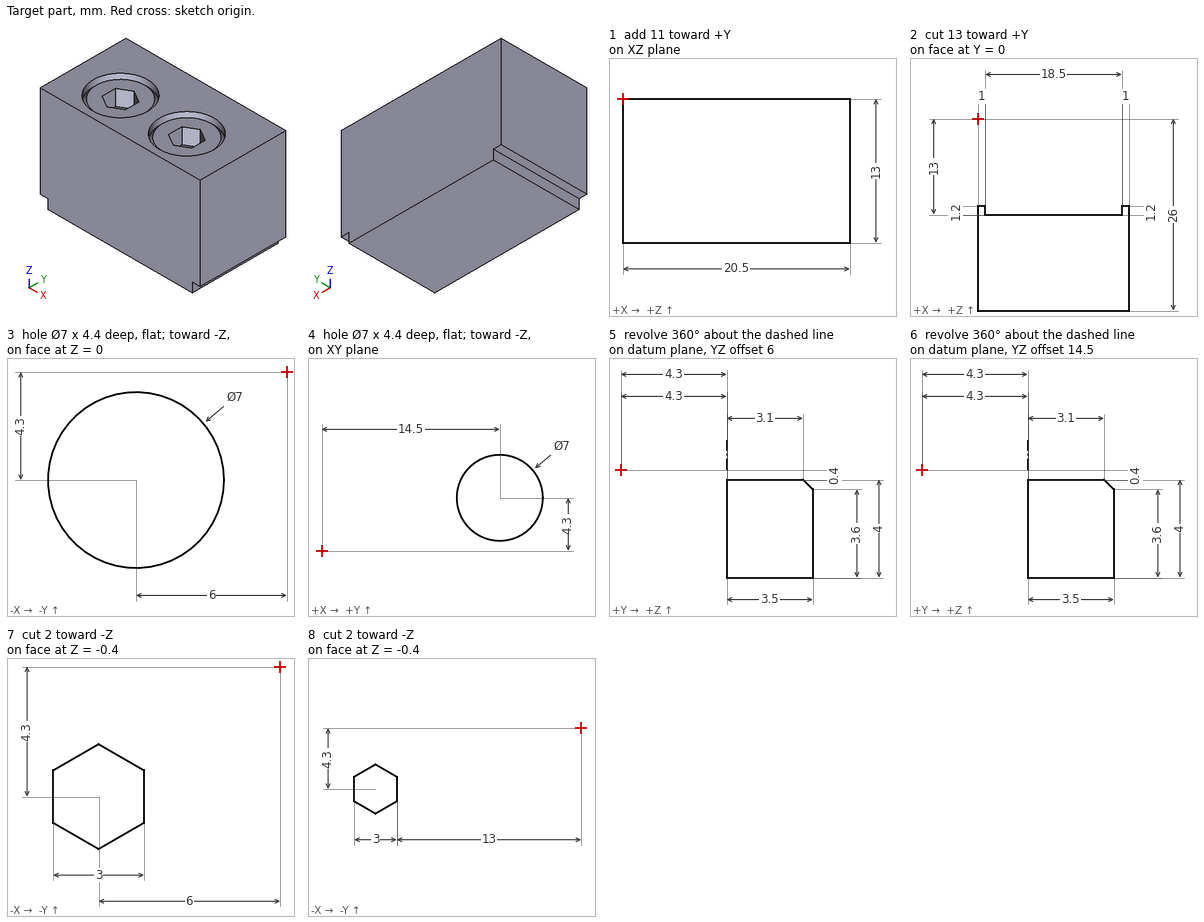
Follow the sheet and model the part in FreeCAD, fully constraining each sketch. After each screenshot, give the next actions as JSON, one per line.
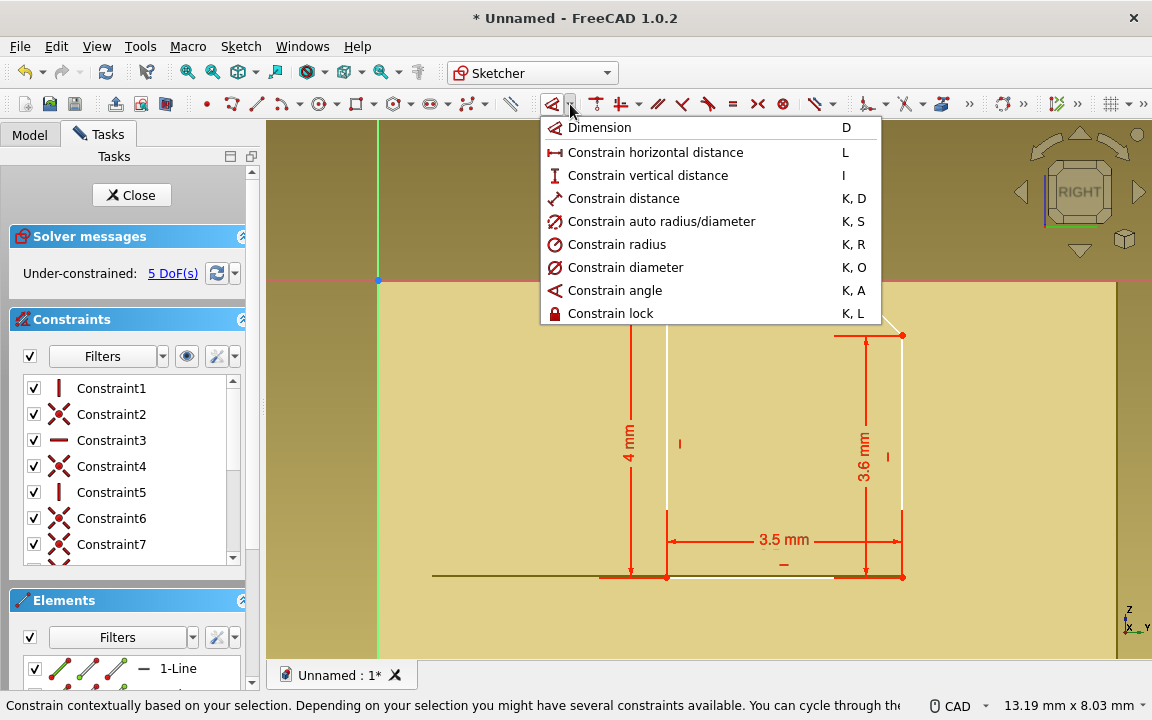
{"action": "left_click", "coordinate": [711, 152]}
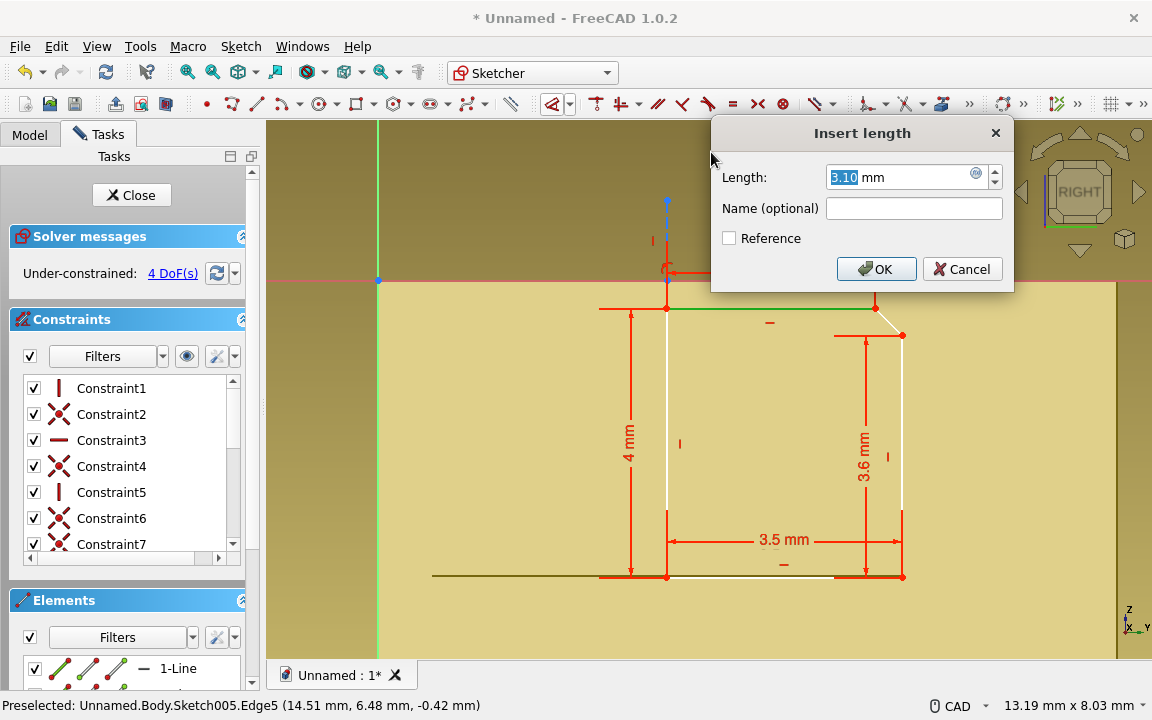
{"action": "type", "text": "3.1"}
{"action": "key", "text": "Return"}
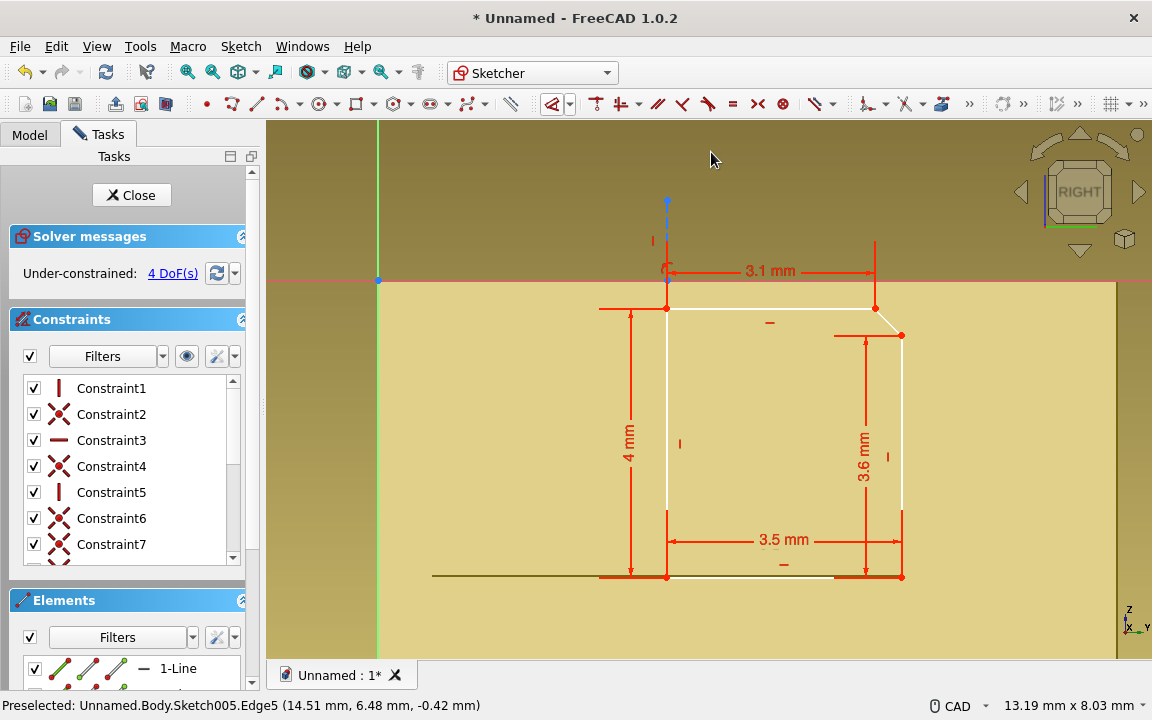
{"action": "left_click", "coordinate": [667, 309]}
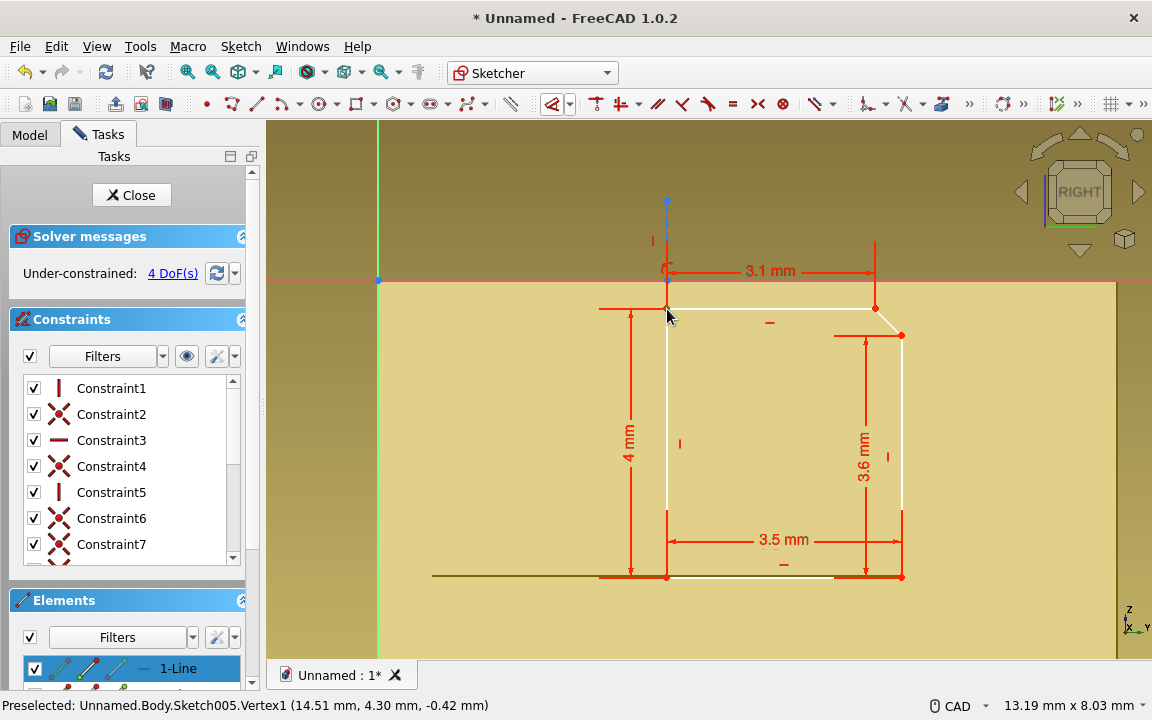
{"action": "key", "text": "l"}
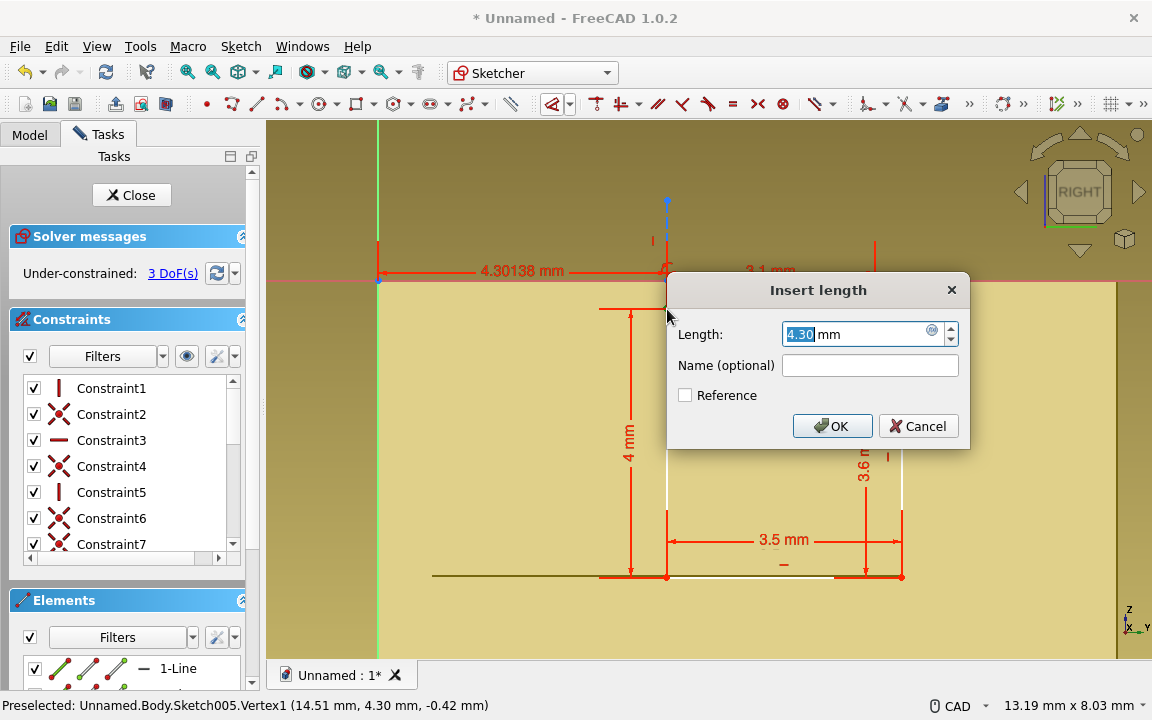
{"action": "type", "text": "4.3"}
{"action": "key", "text": "Return"}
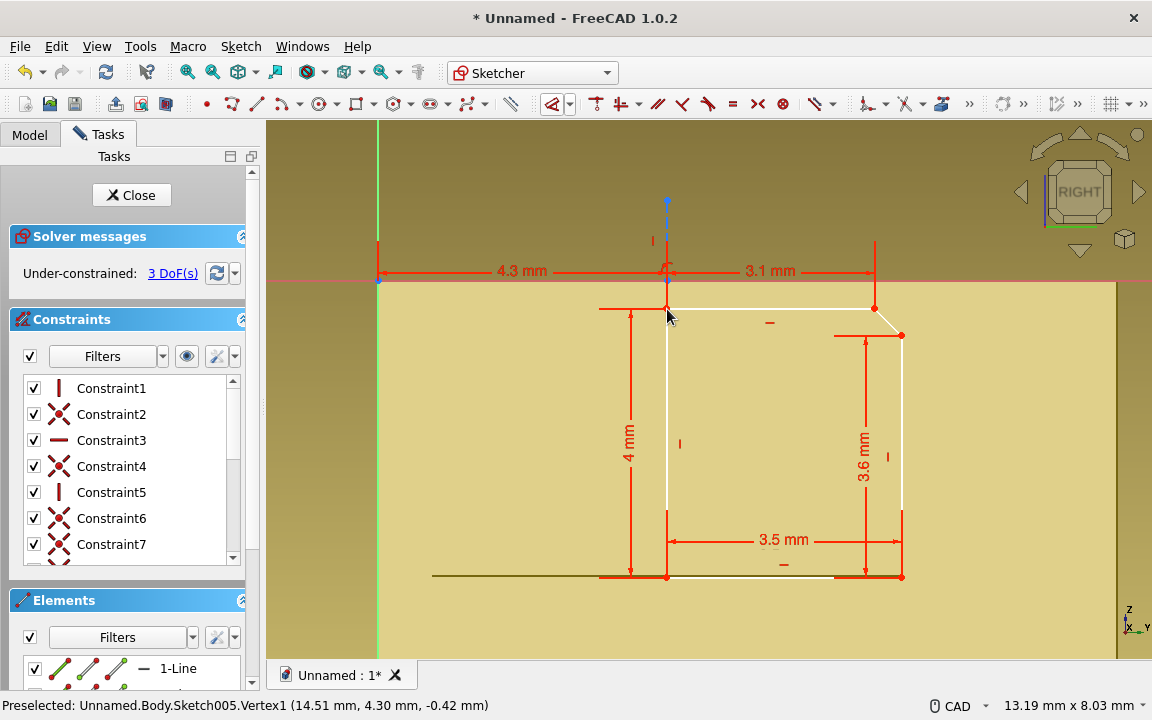
{"action": "scroll", "coordinate": [667, 309], "scroll_direction": "up", "scroll_amount": 2}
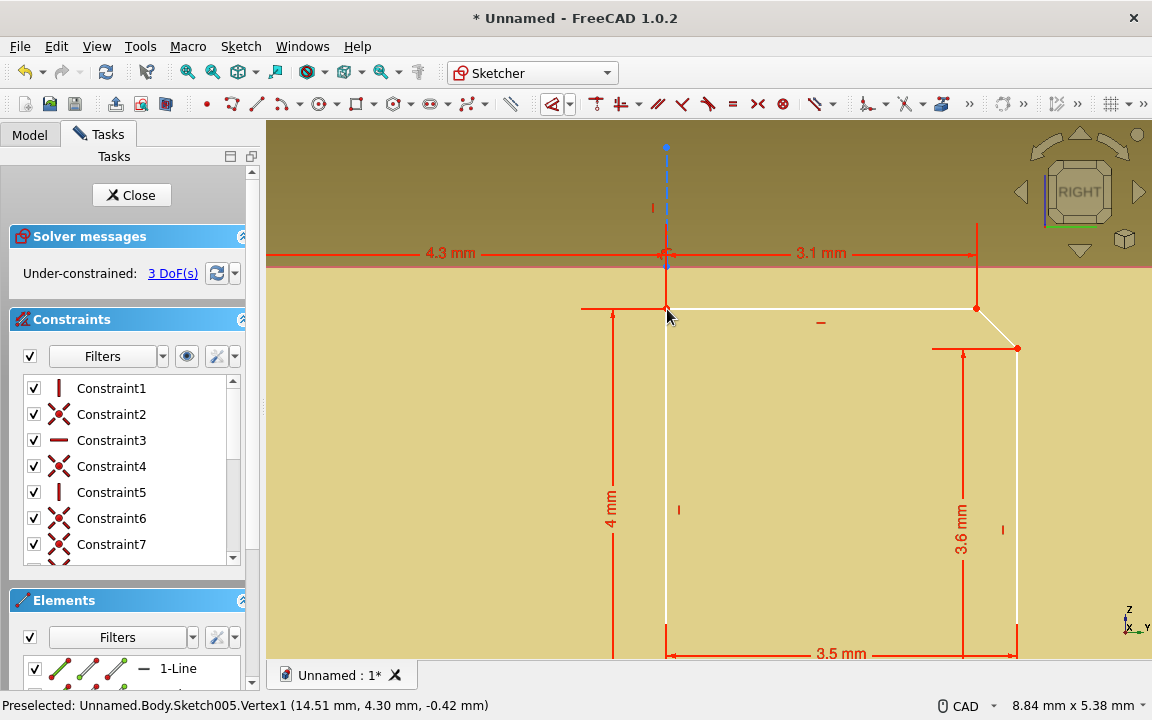
{"action": "left_click", "coordinate": [666, 309]}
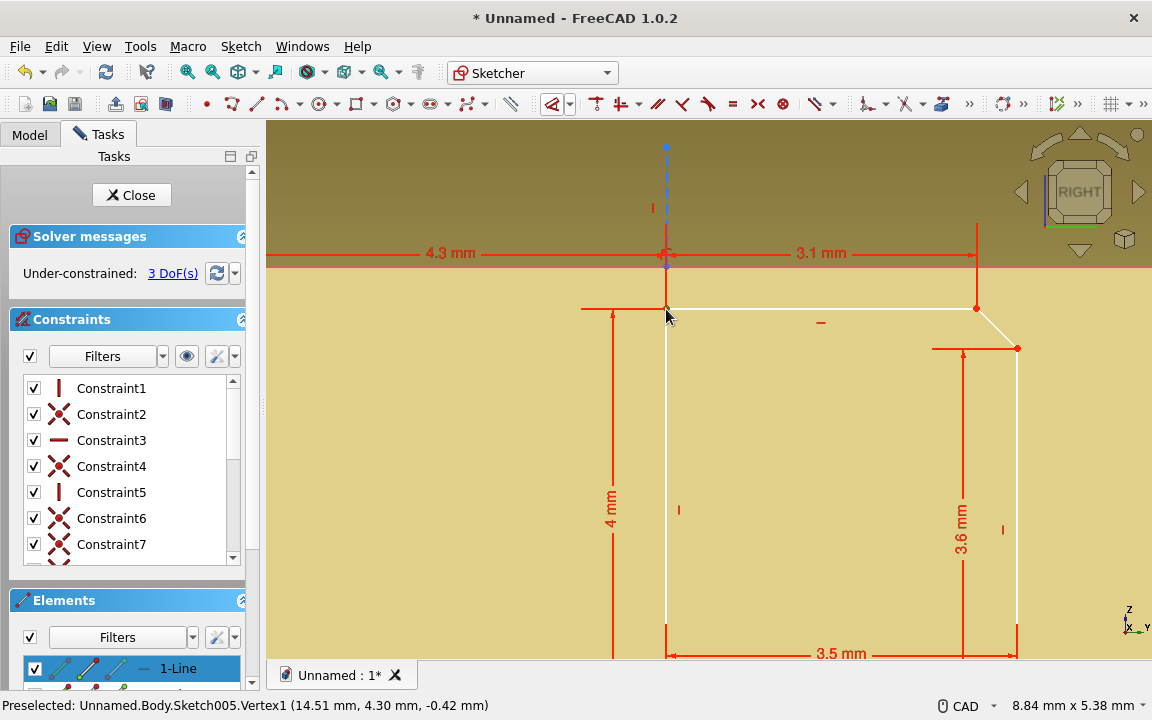
{"action": "left_click", "coordinate": [570, 104]}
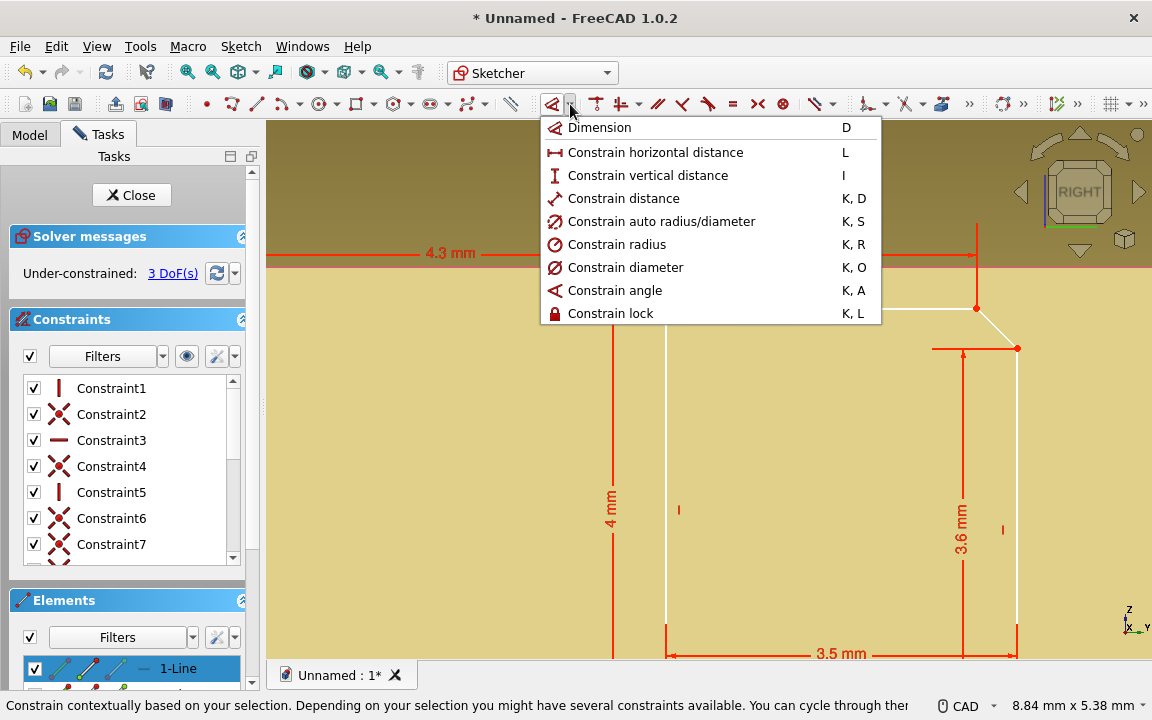
{"action": "left_click", "coordinate": [711, 176]}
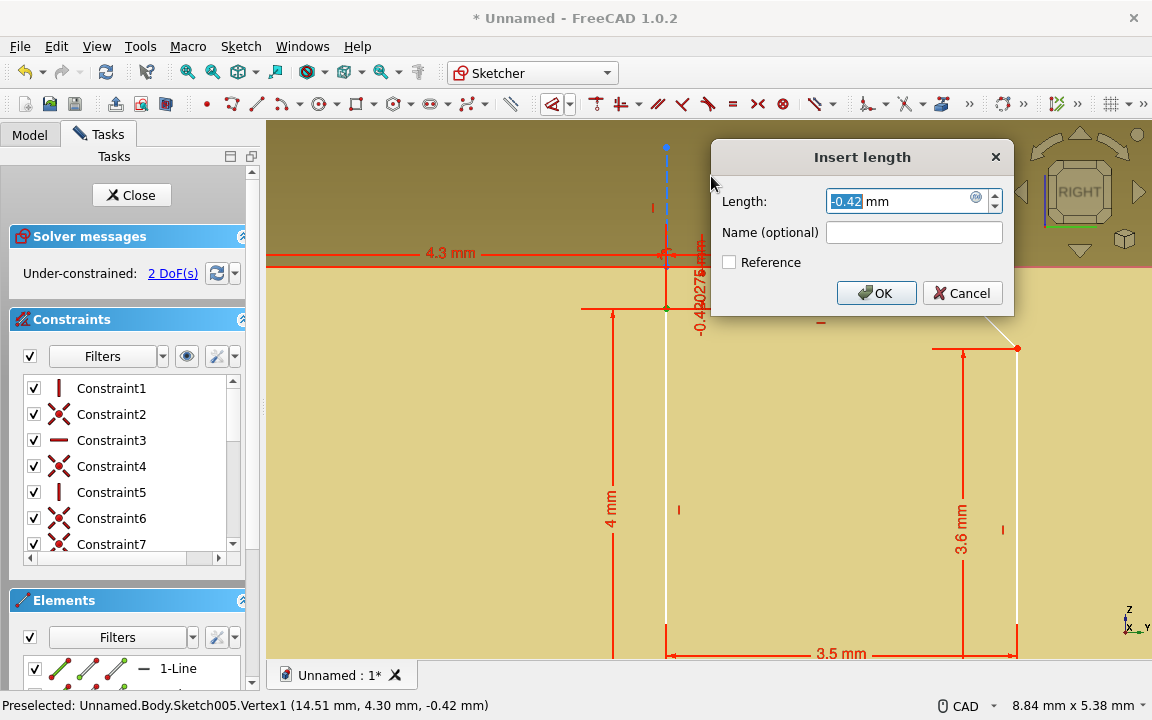
{"action": "type", "text": "-0.4"}
{"action": "key", "text": "Return"}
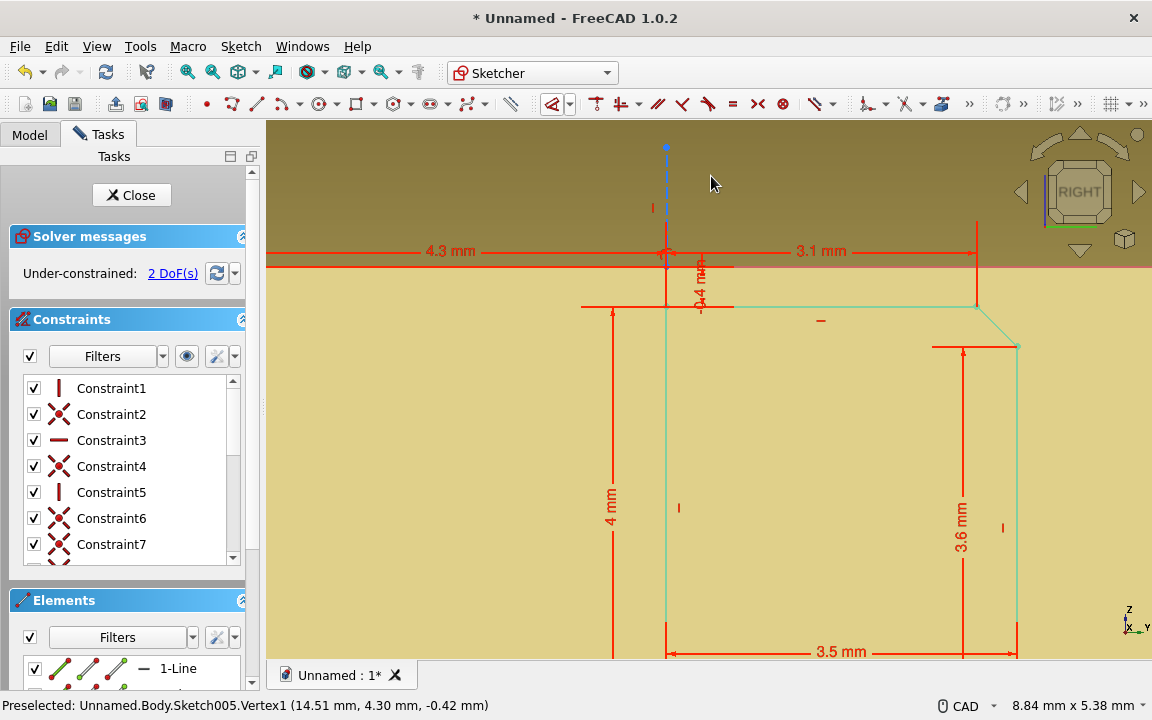
{"action": "left_click", "coordinate": [667, 267]}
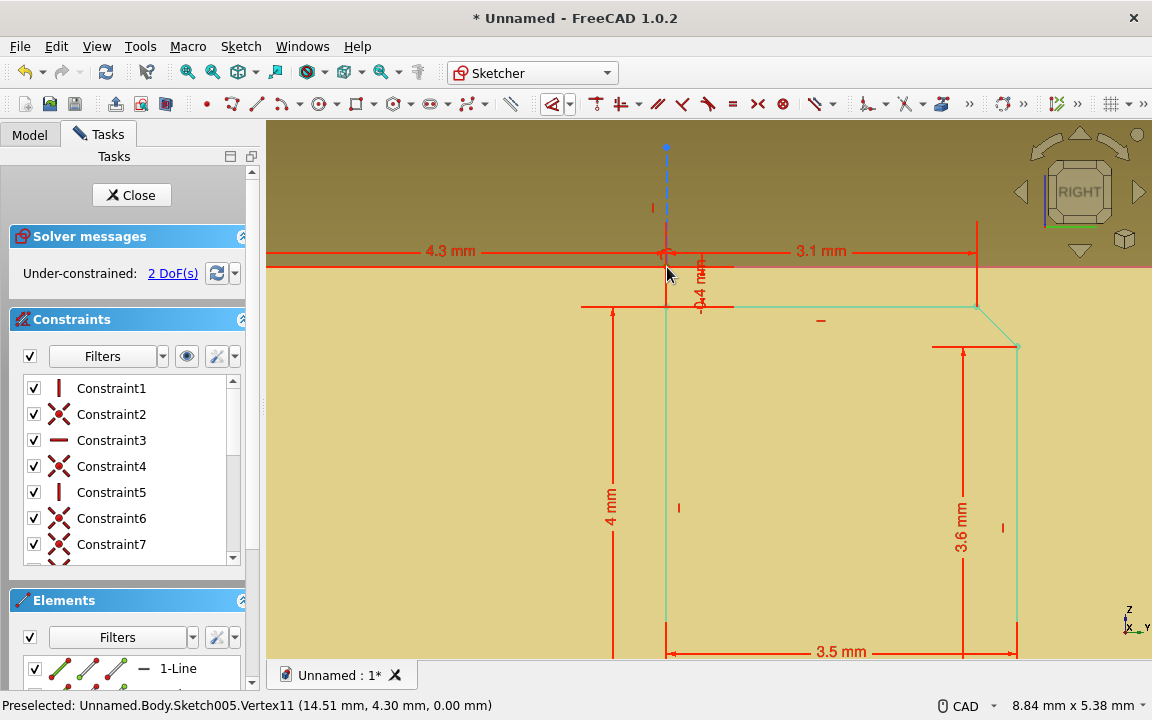
{"action": "key", "text": "l"}